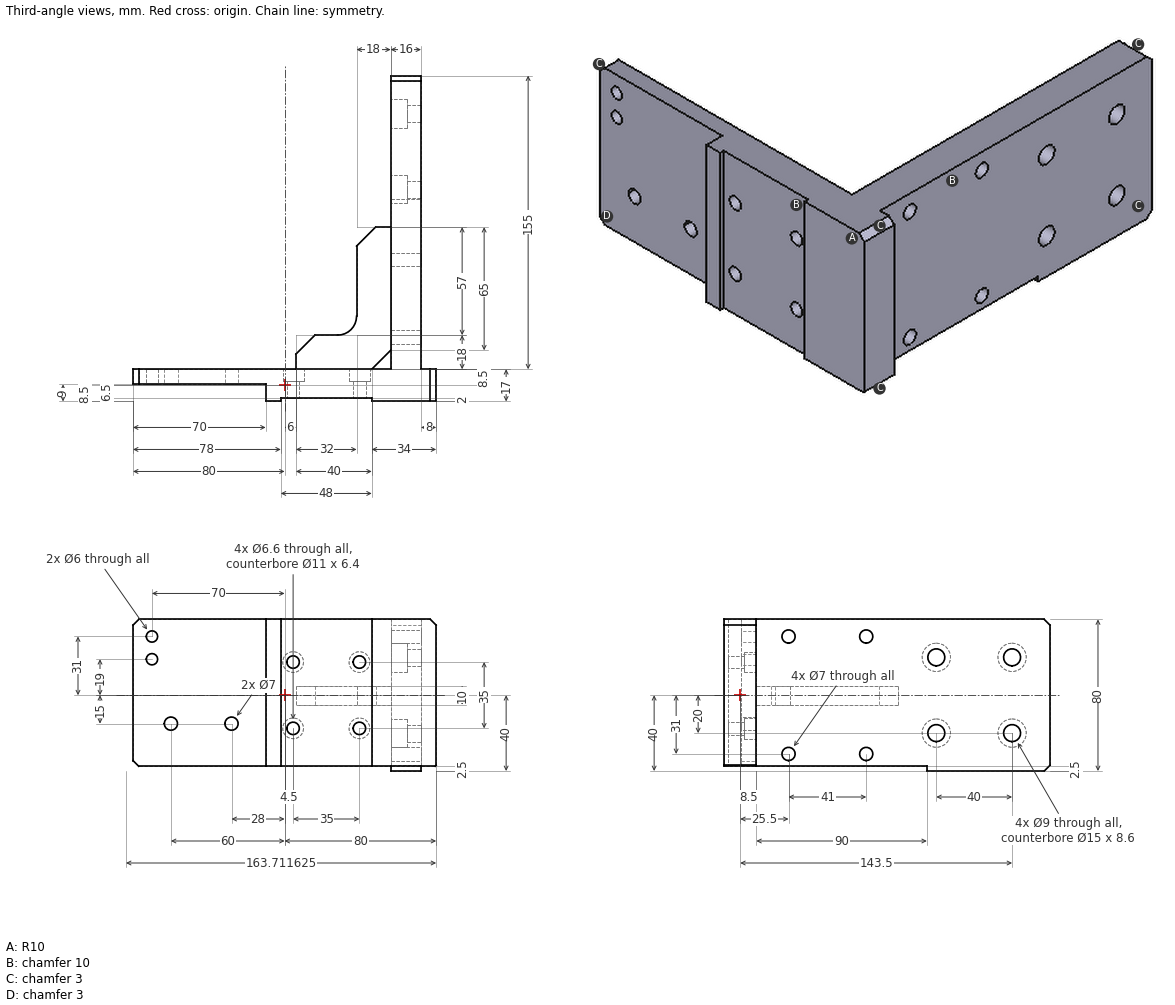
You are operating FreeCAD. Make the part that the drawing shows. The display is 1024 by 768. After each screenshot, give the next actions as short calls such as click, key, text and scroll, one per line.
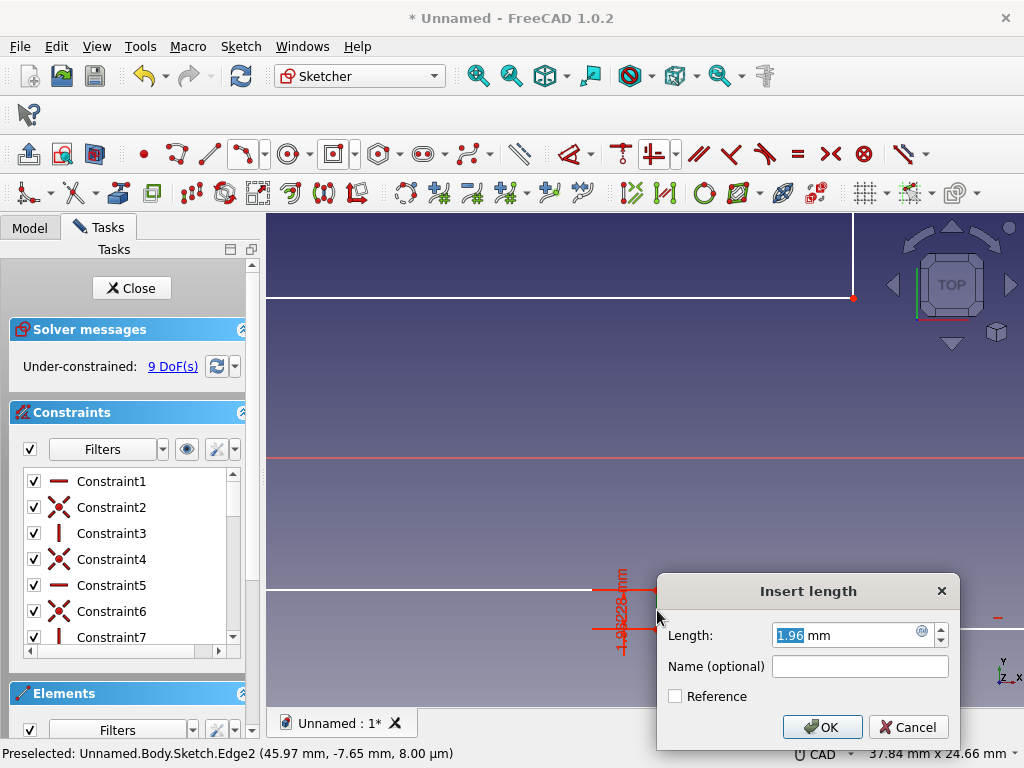
text(2)
key(Return)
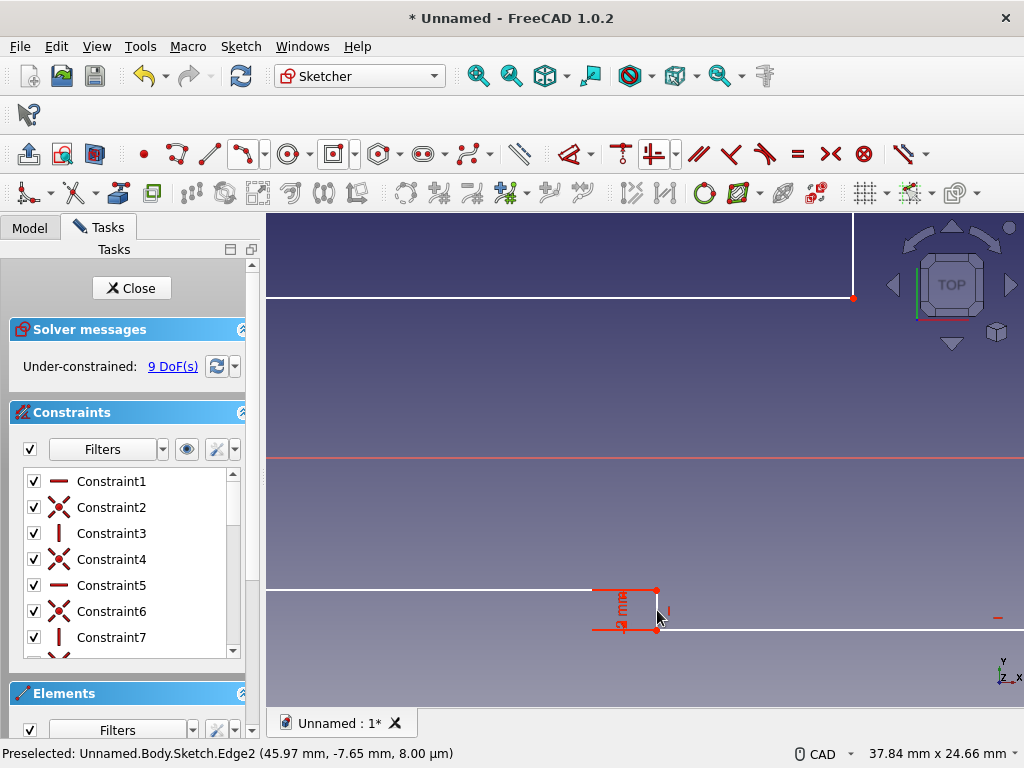
scroll(660, 615, down, 12)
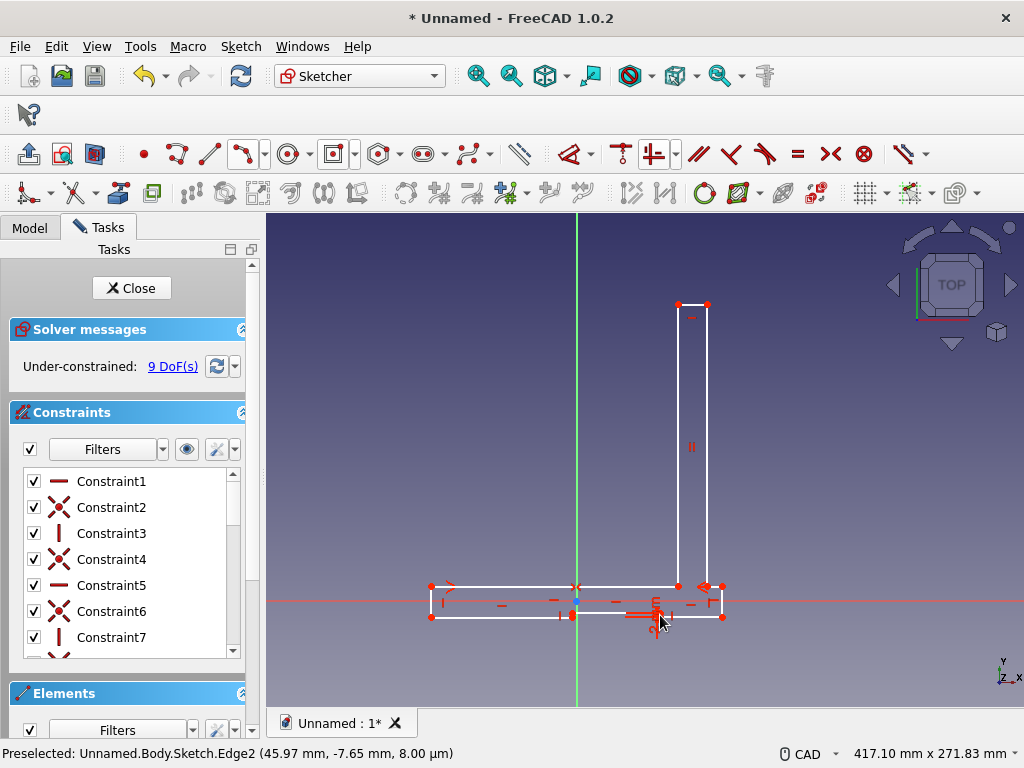
scroll(718, 587, up, 6)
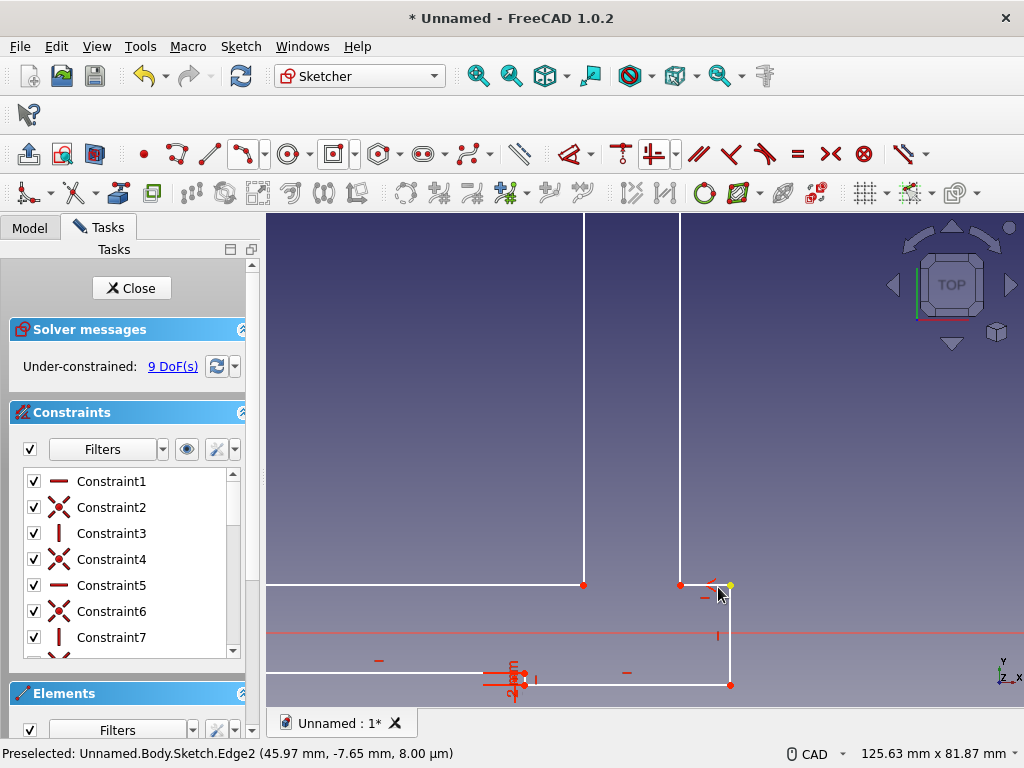
click(715, 585)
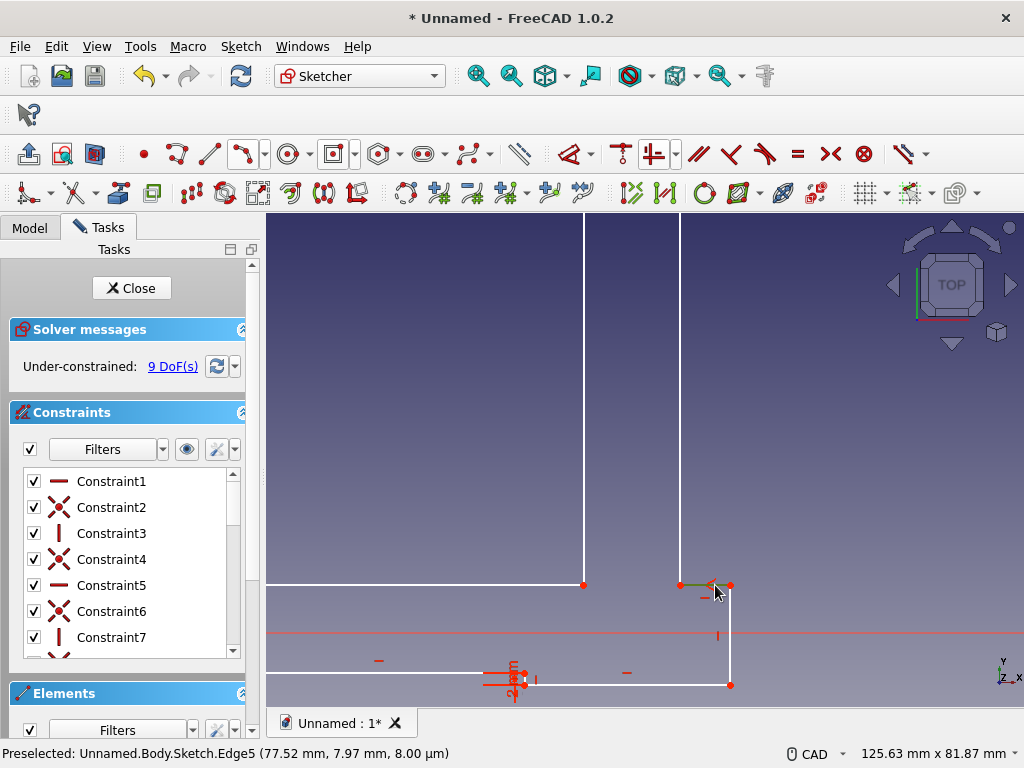
click(590, 154)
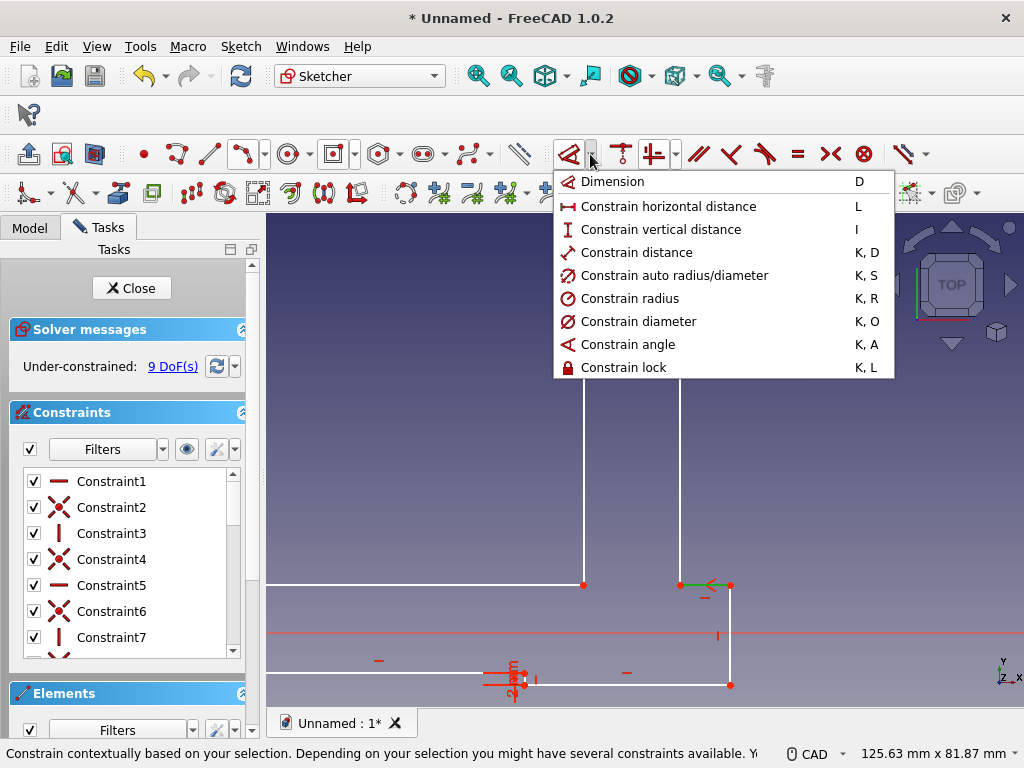
click(724, 206)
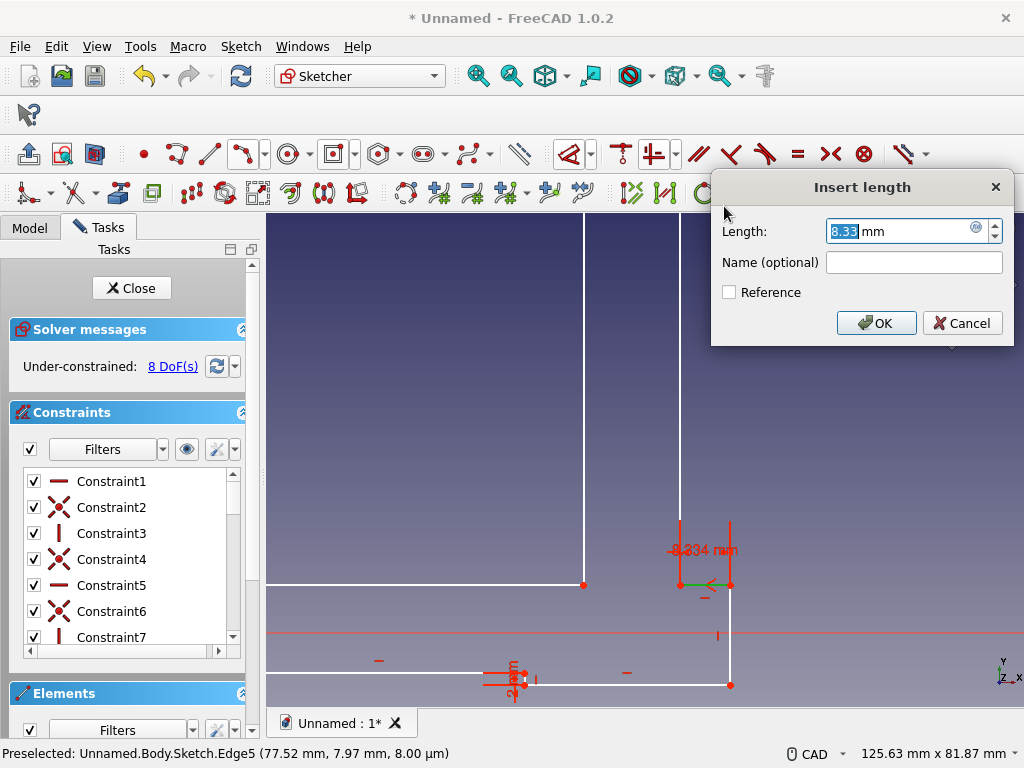
text(8)
key(Return)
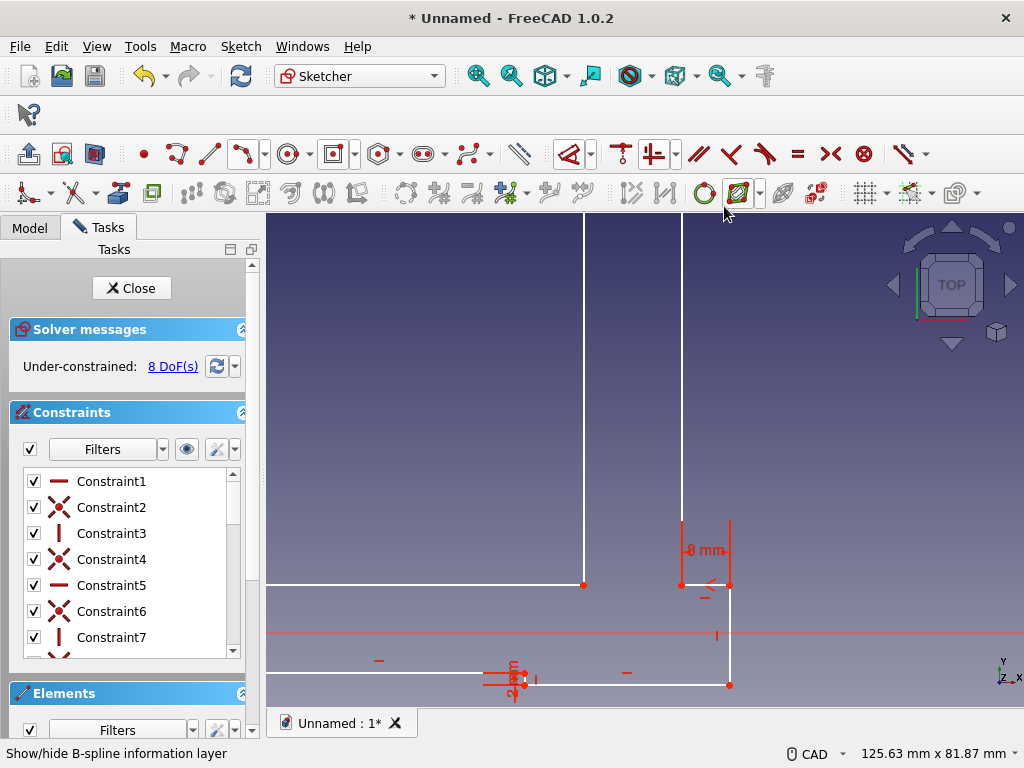
scroll(718, 587, down, 6)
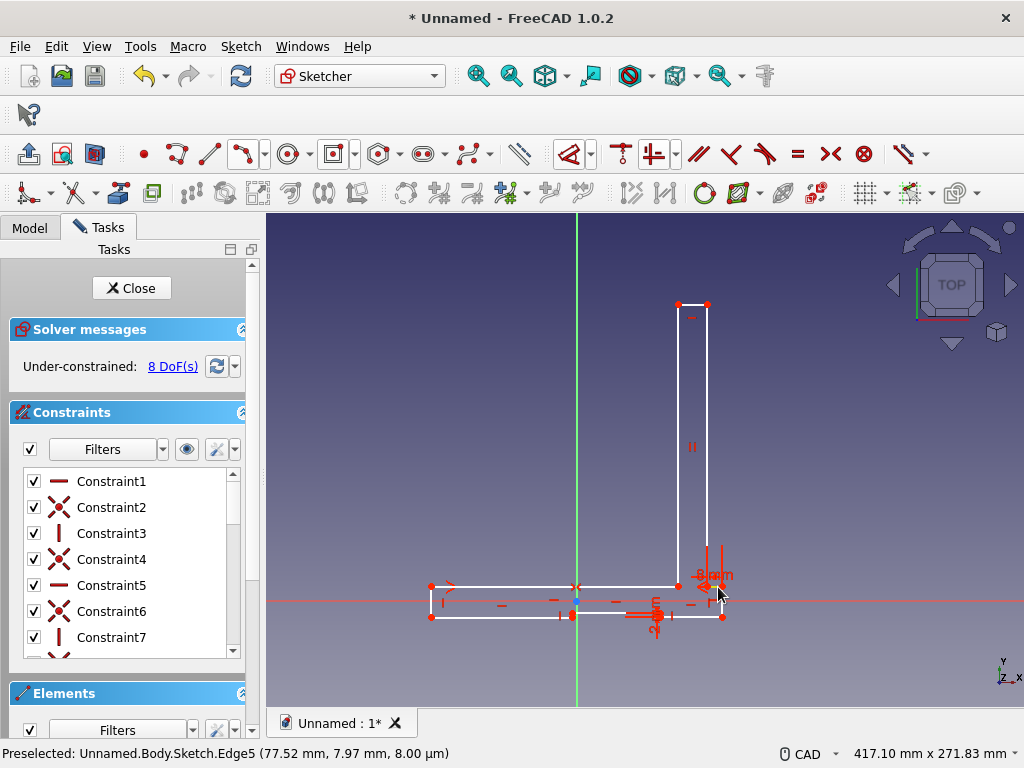
scroll(573, 616, up, 12)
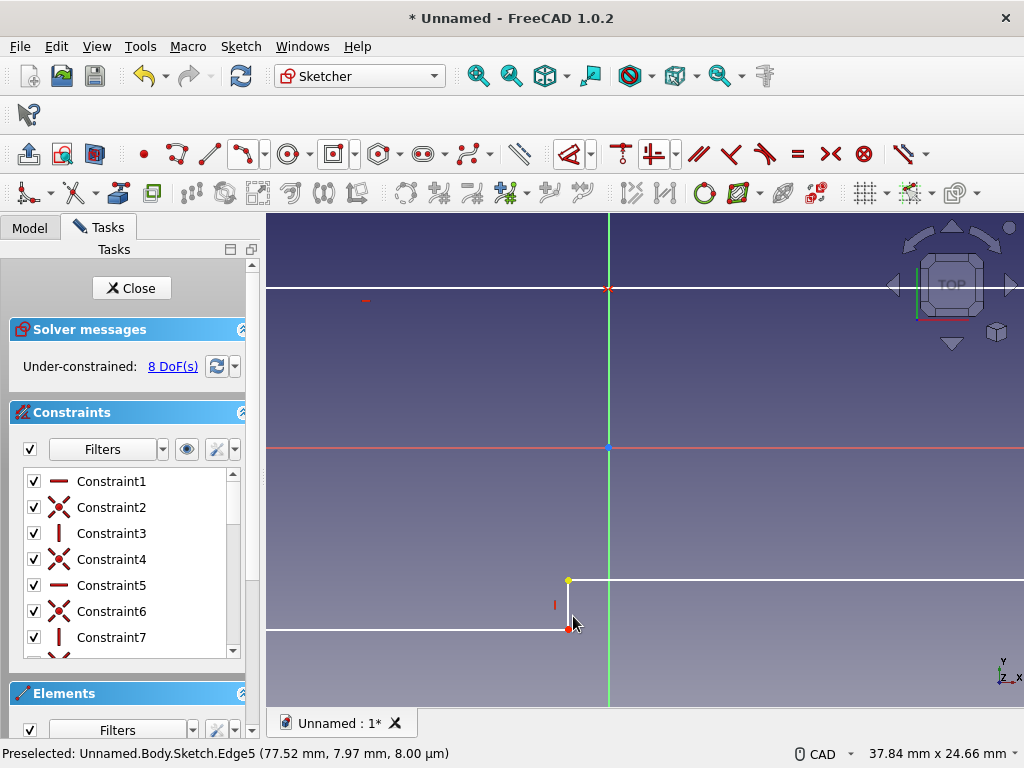
click(568, 605)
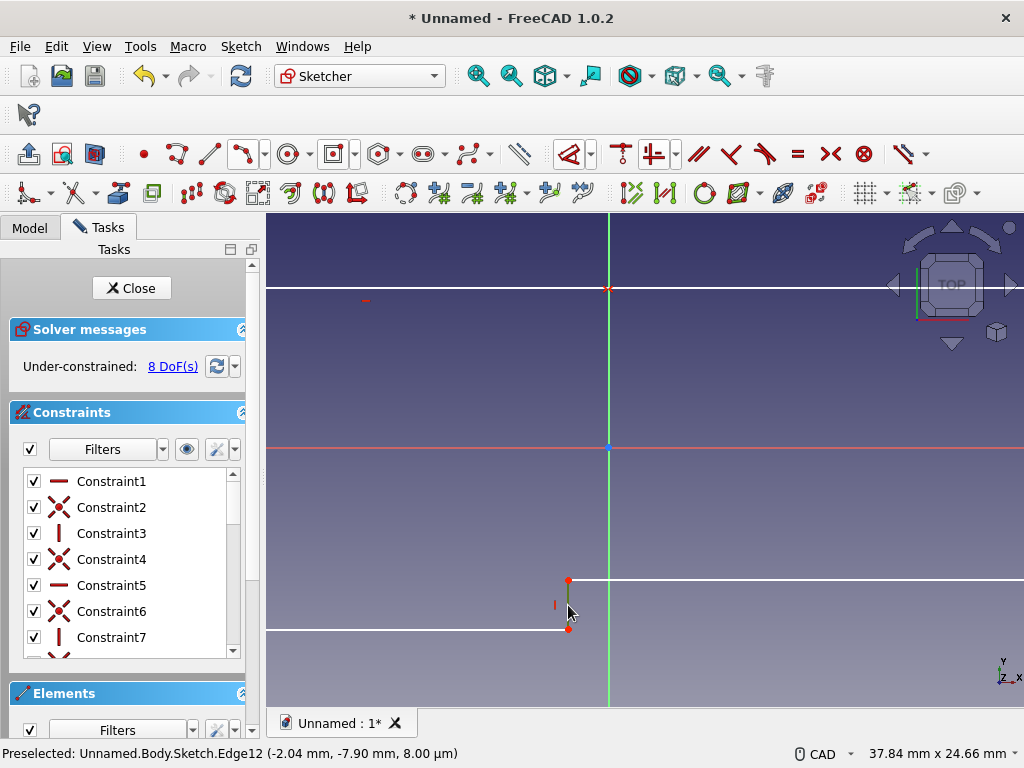
key(i)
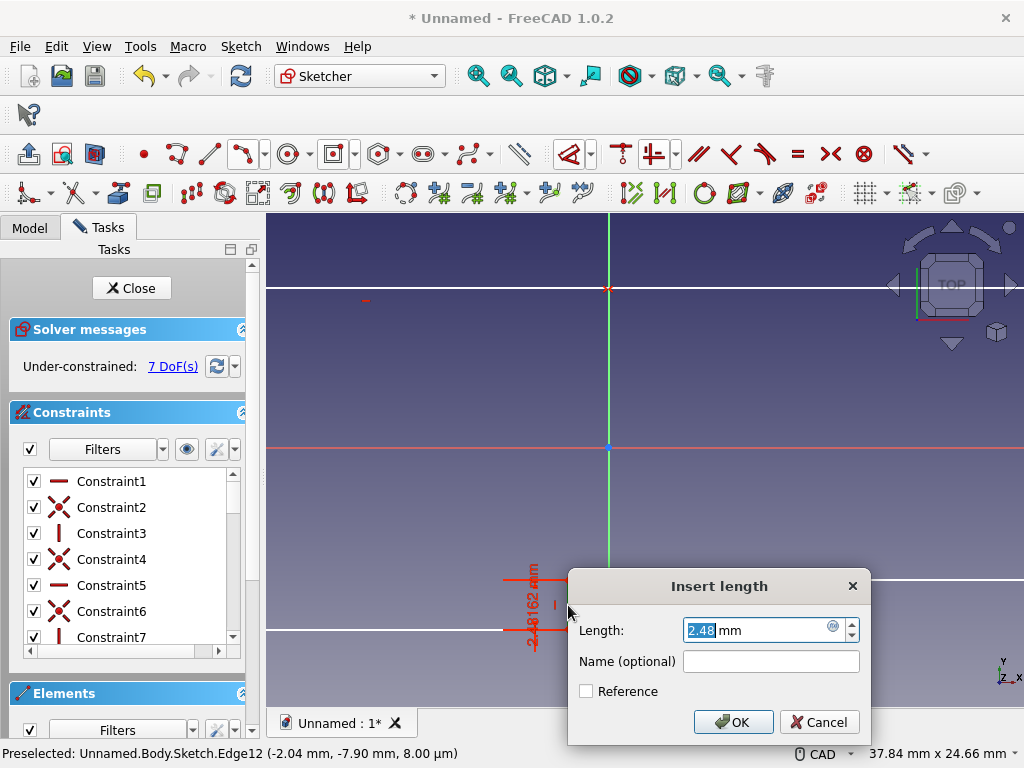
text(2)
key(Return)